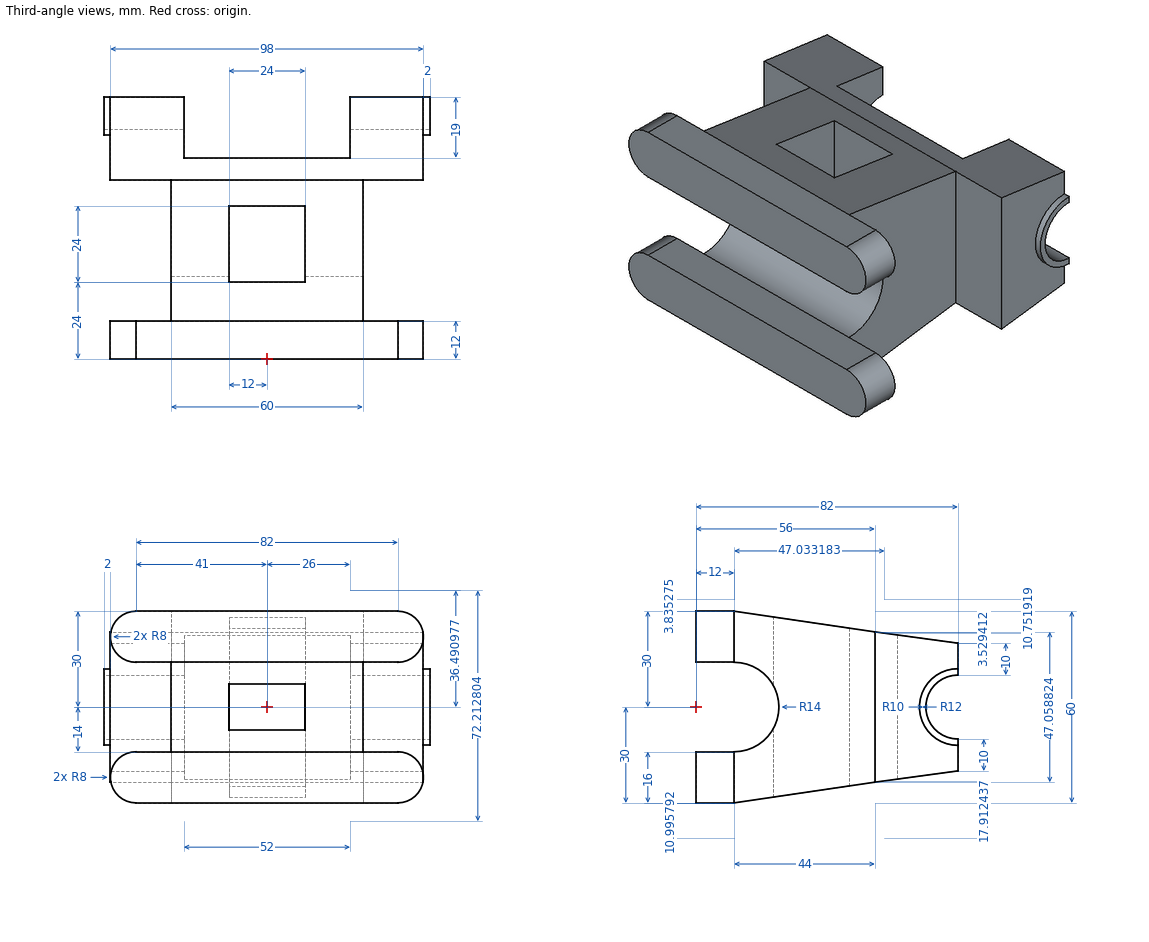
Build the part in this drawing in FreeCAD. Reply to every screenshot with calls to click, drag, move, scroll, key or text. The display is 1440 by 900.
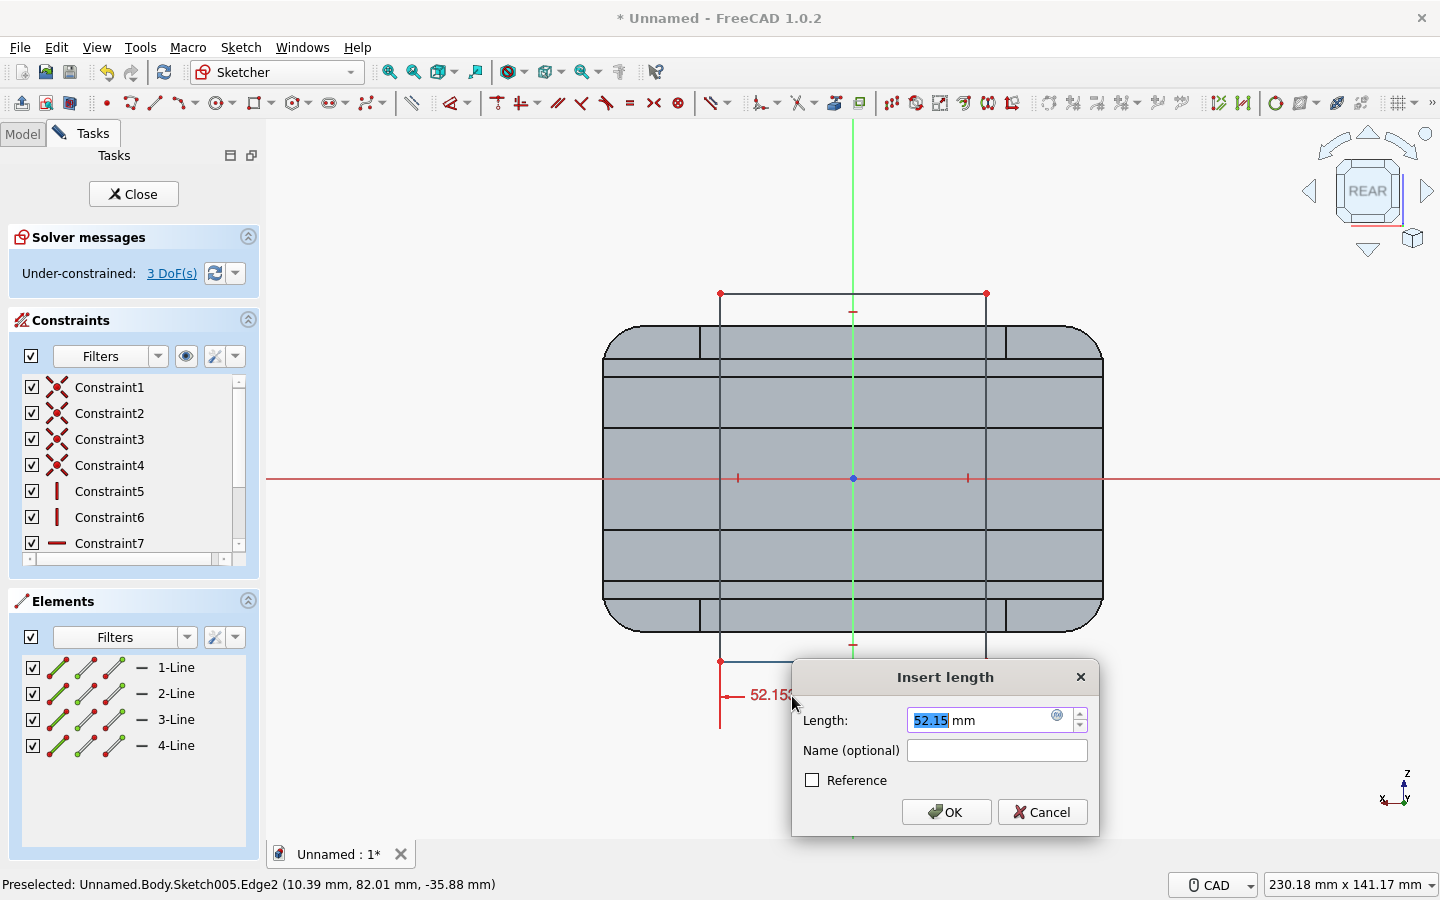
text(52)
key(Return)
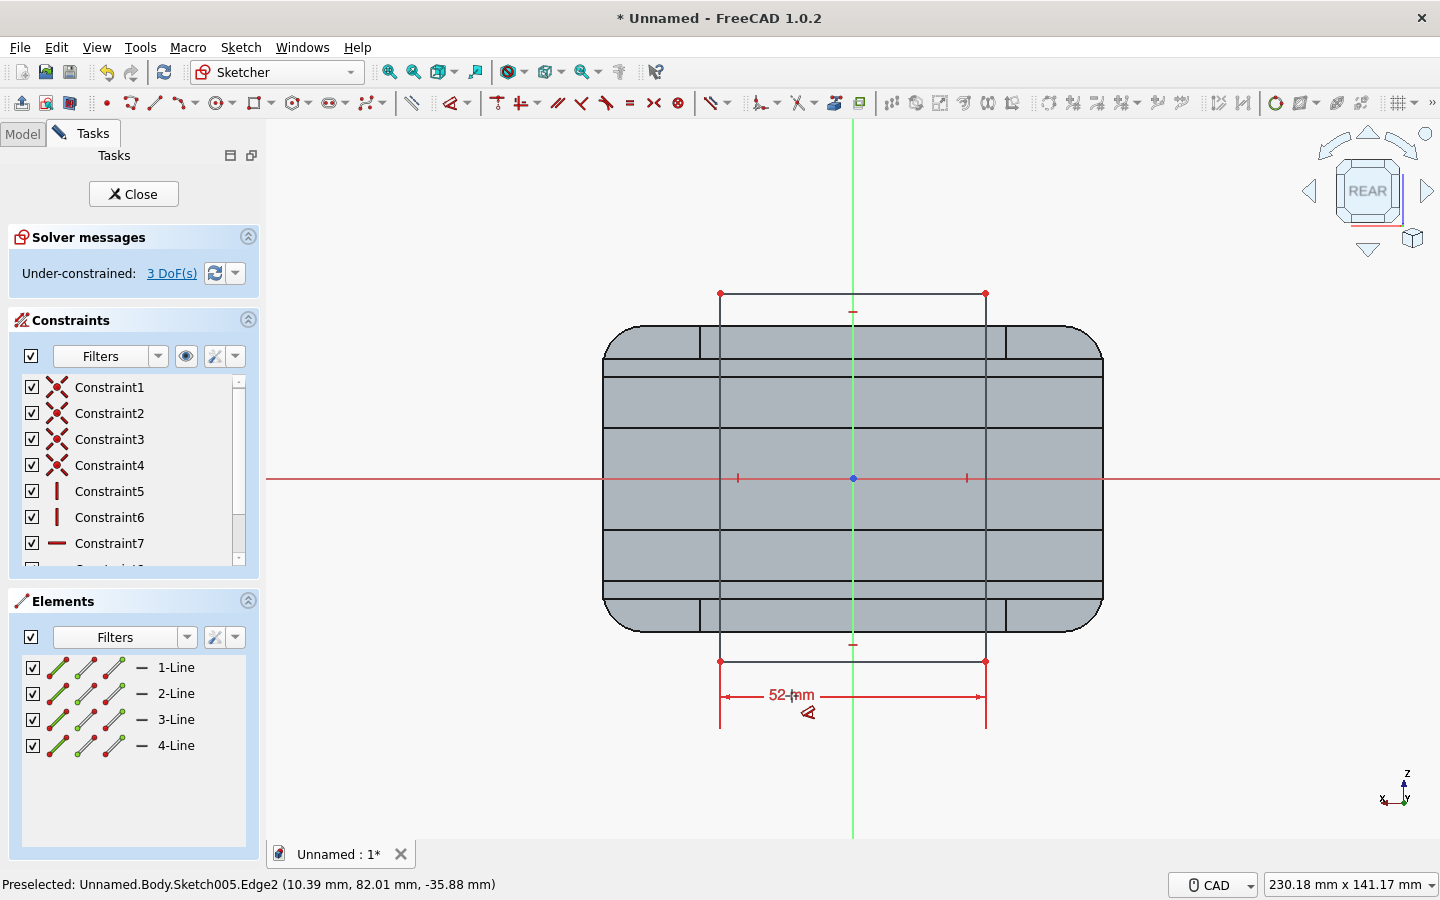
click(720, 294)
click(787, 260)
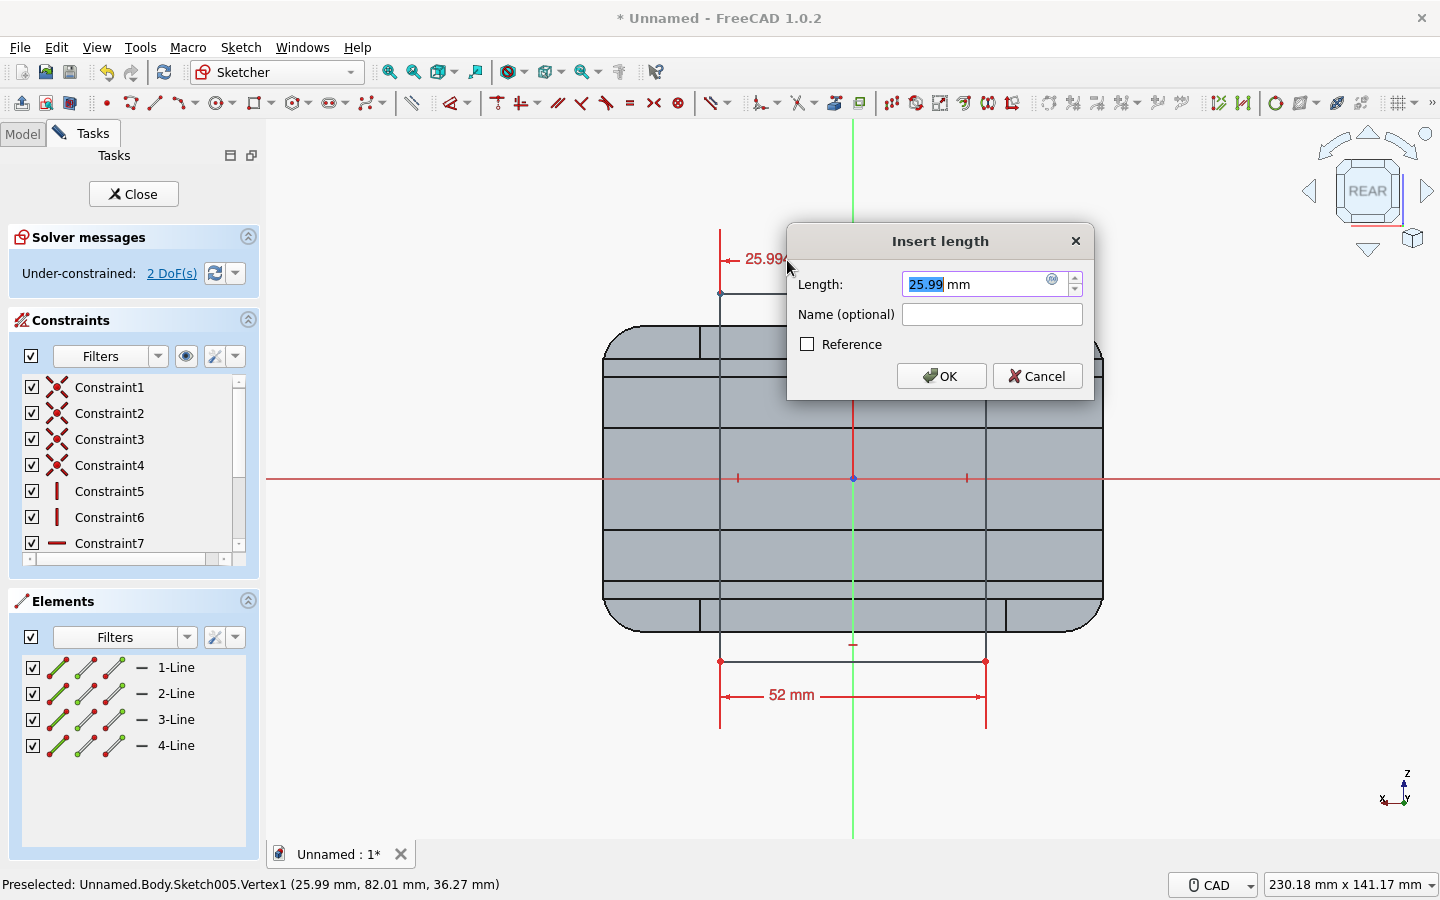
text(26)
key(Return)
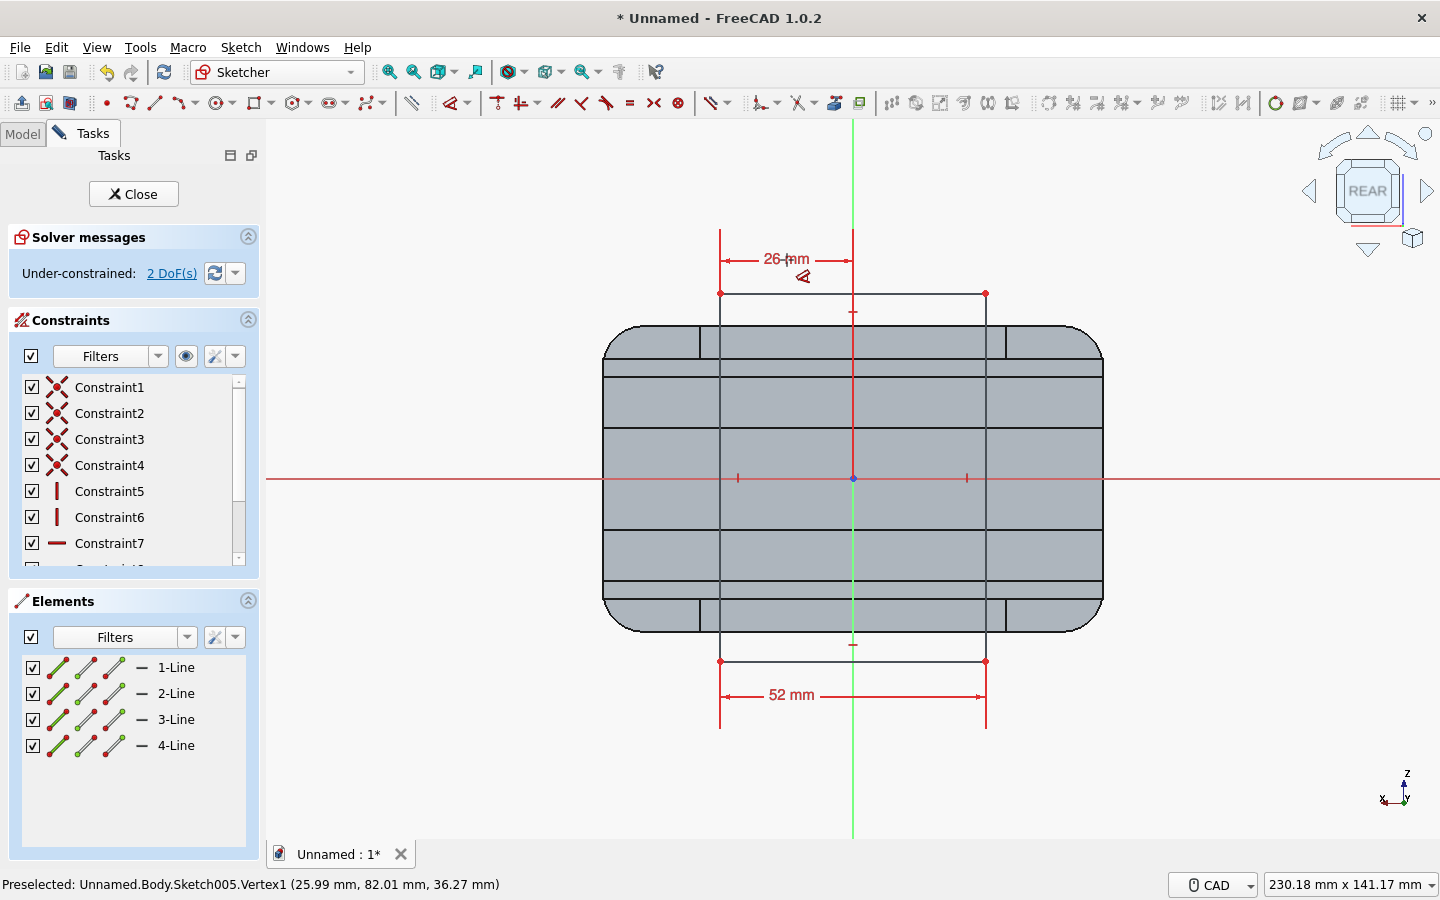
click(720, 404)
click(686, 393)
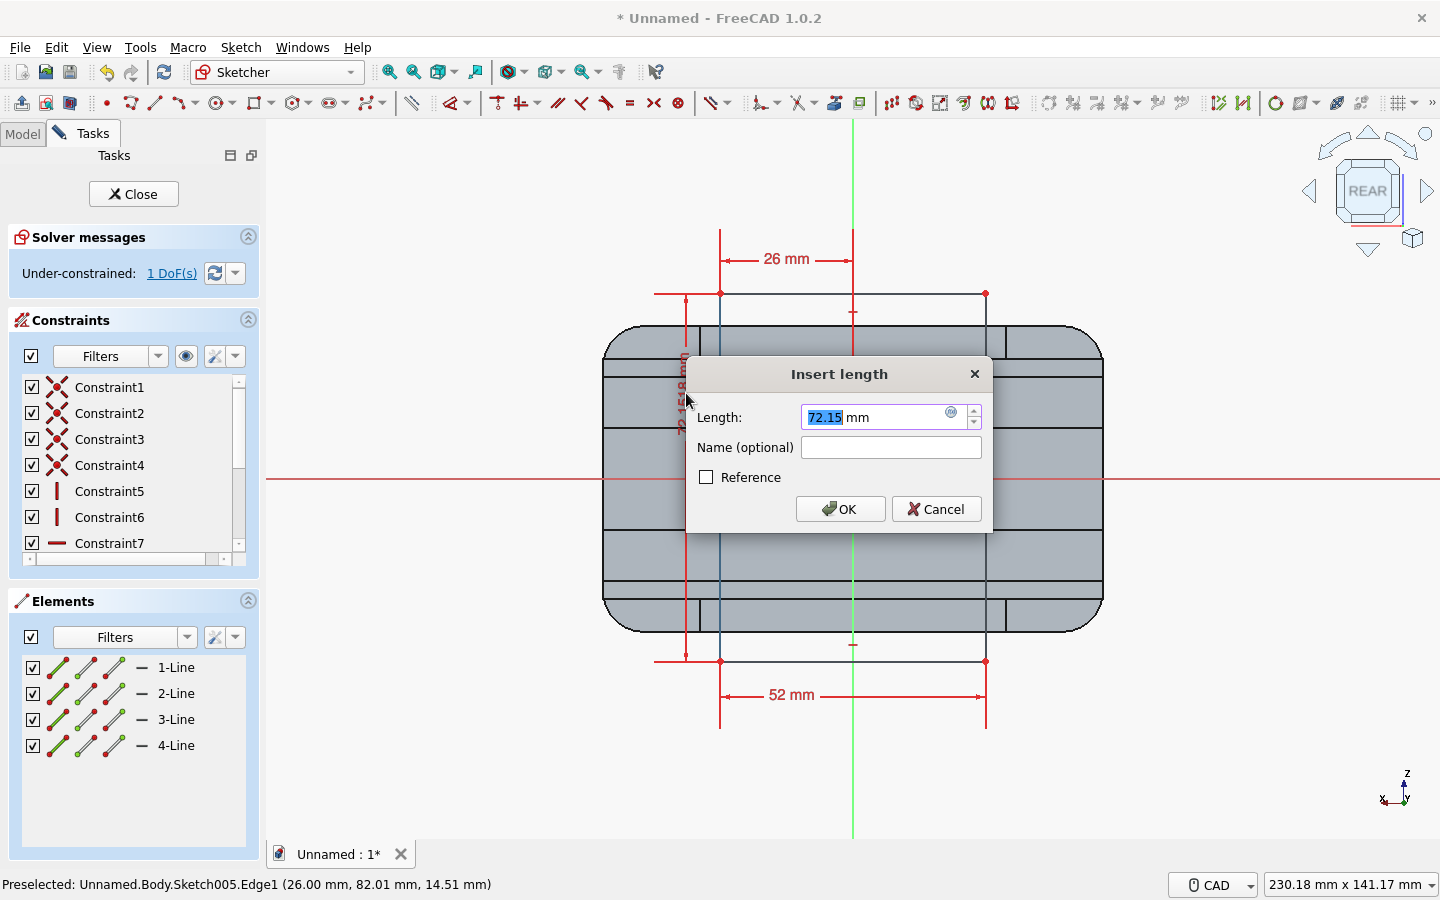
text(72.212804)
key(Return)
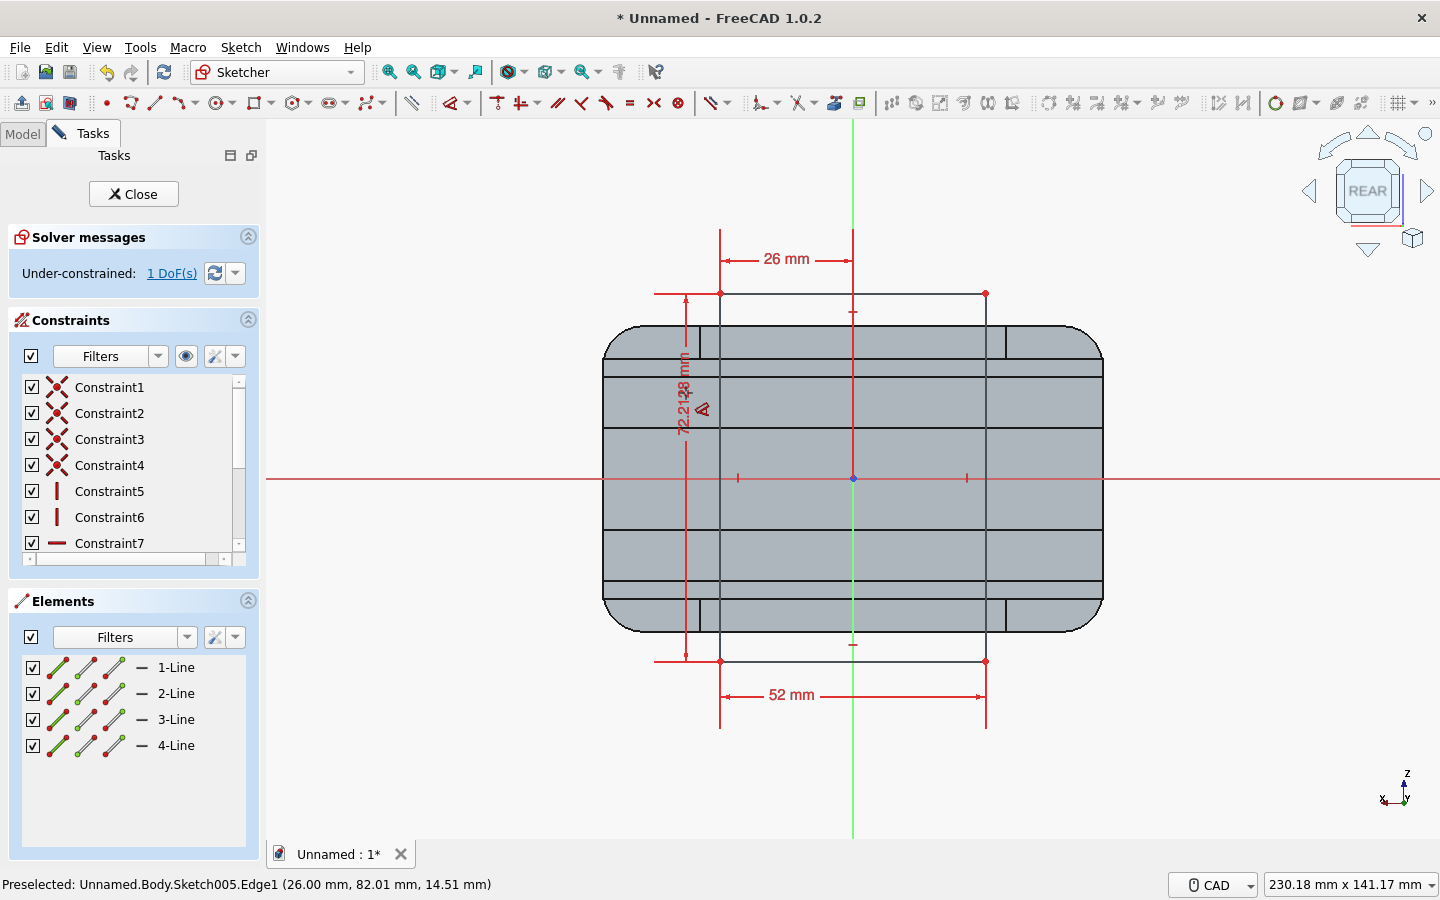
click(720, 294)
click(686, 344)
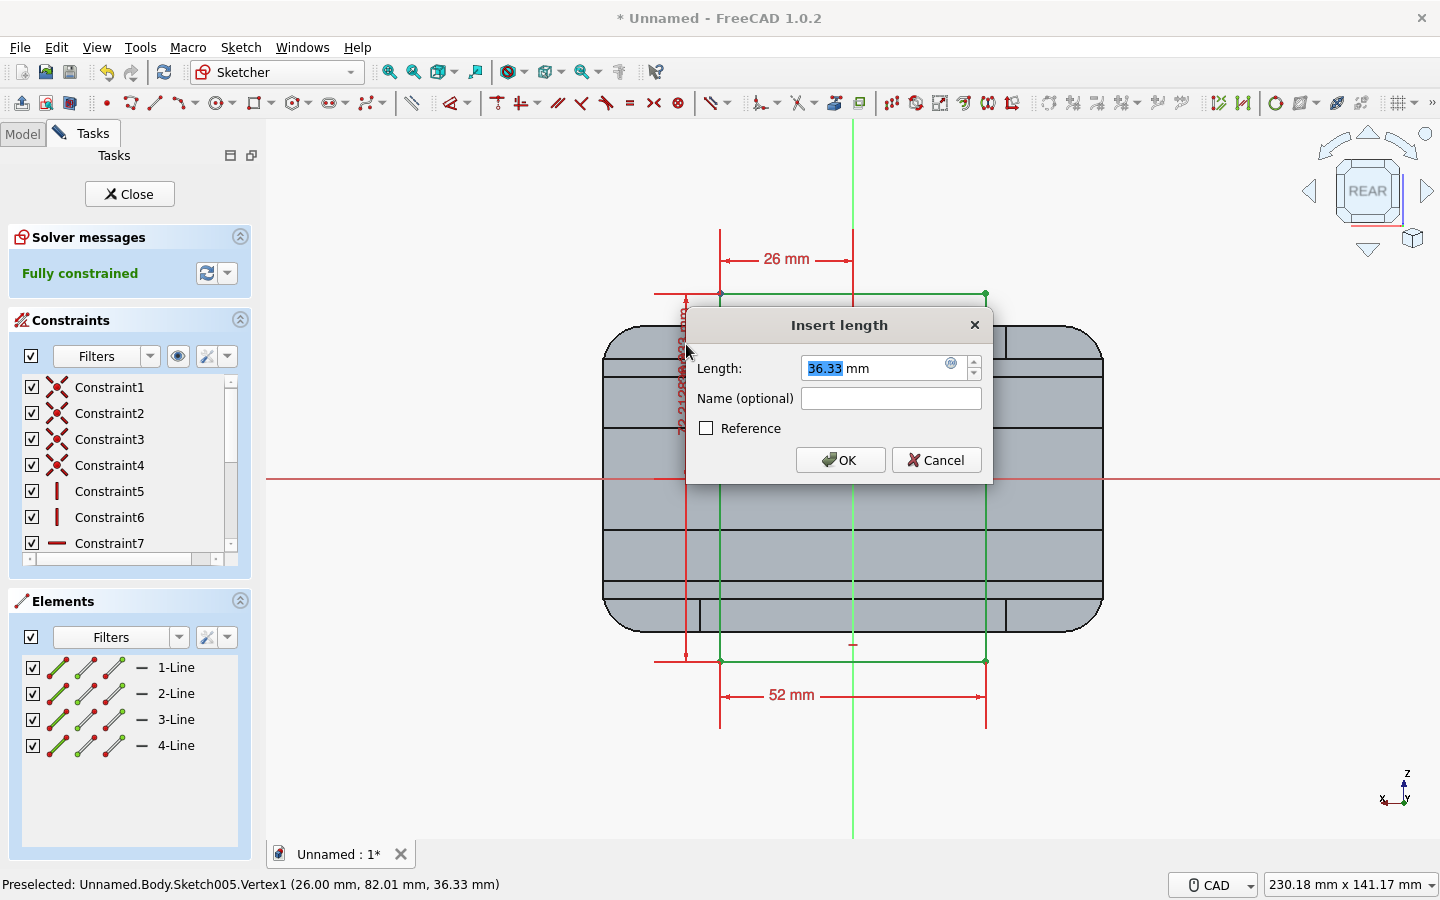
text(36.490977)
key(Return)
key(Escape)